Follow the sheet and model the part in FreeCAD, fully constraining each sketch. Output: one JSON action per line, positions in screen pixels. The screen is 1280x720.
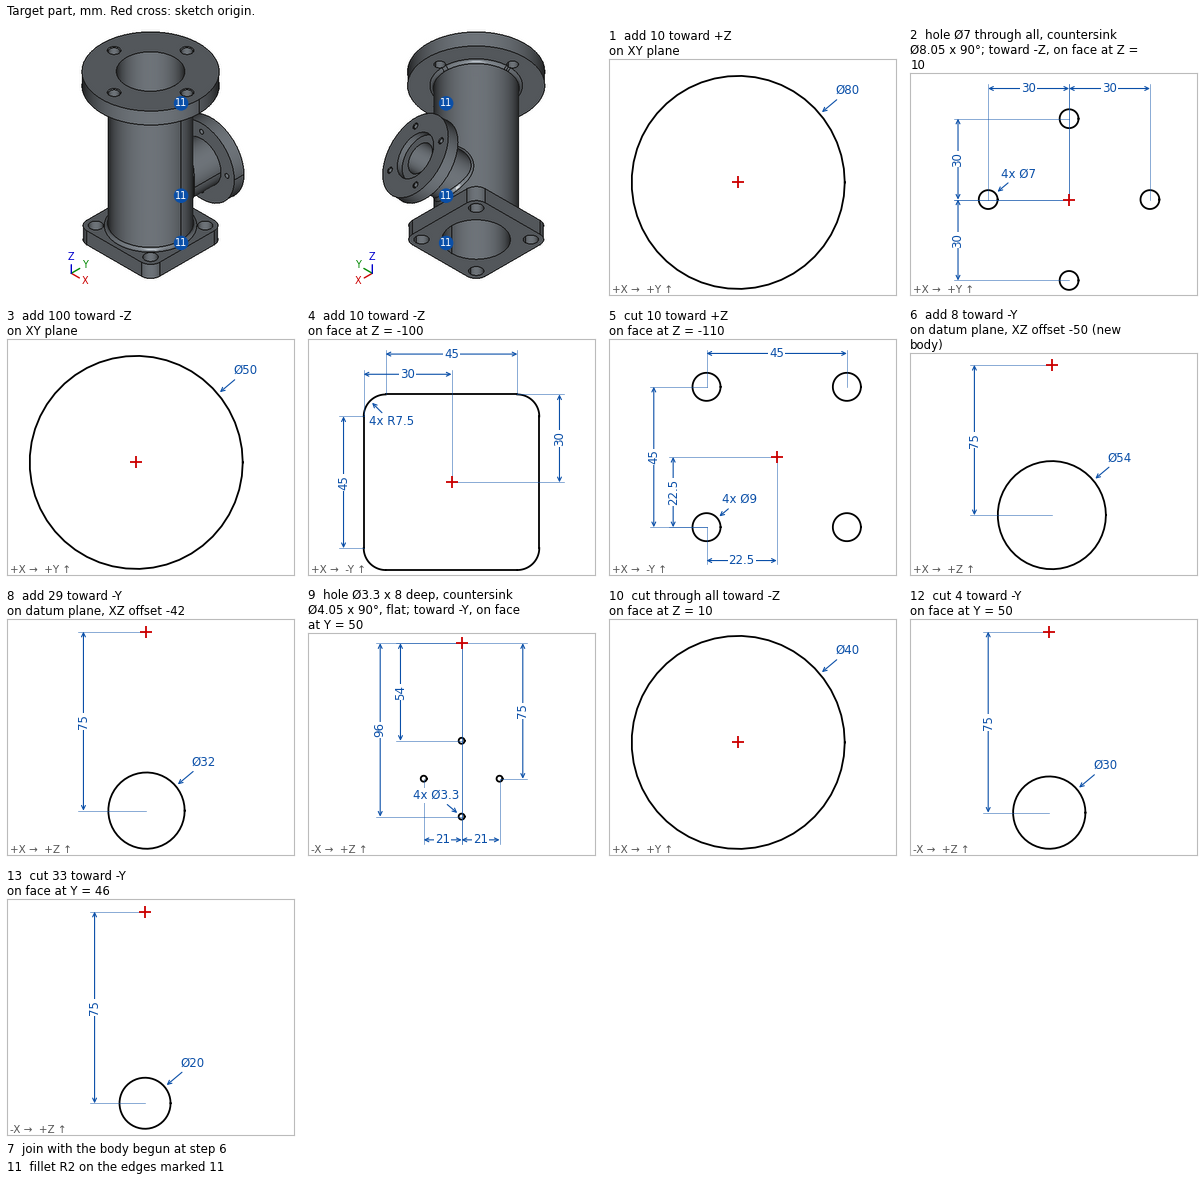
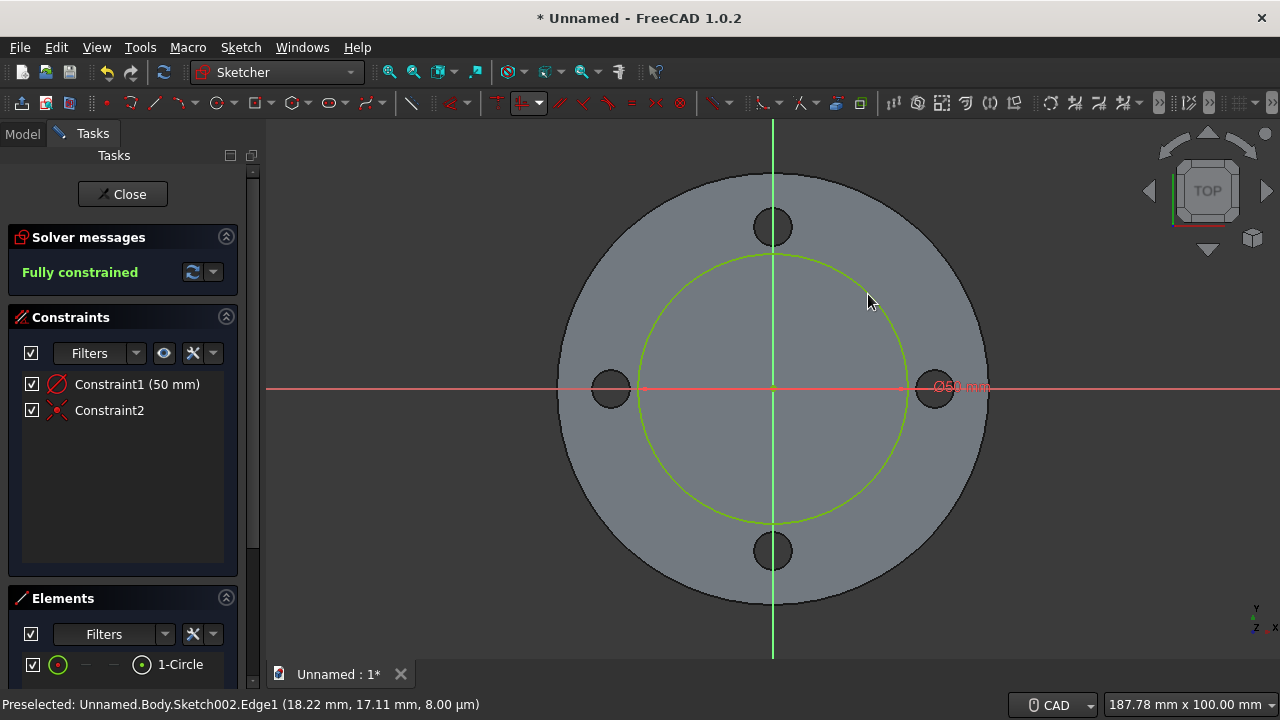
{"action": "left_click", "coordinate": [123, 194]}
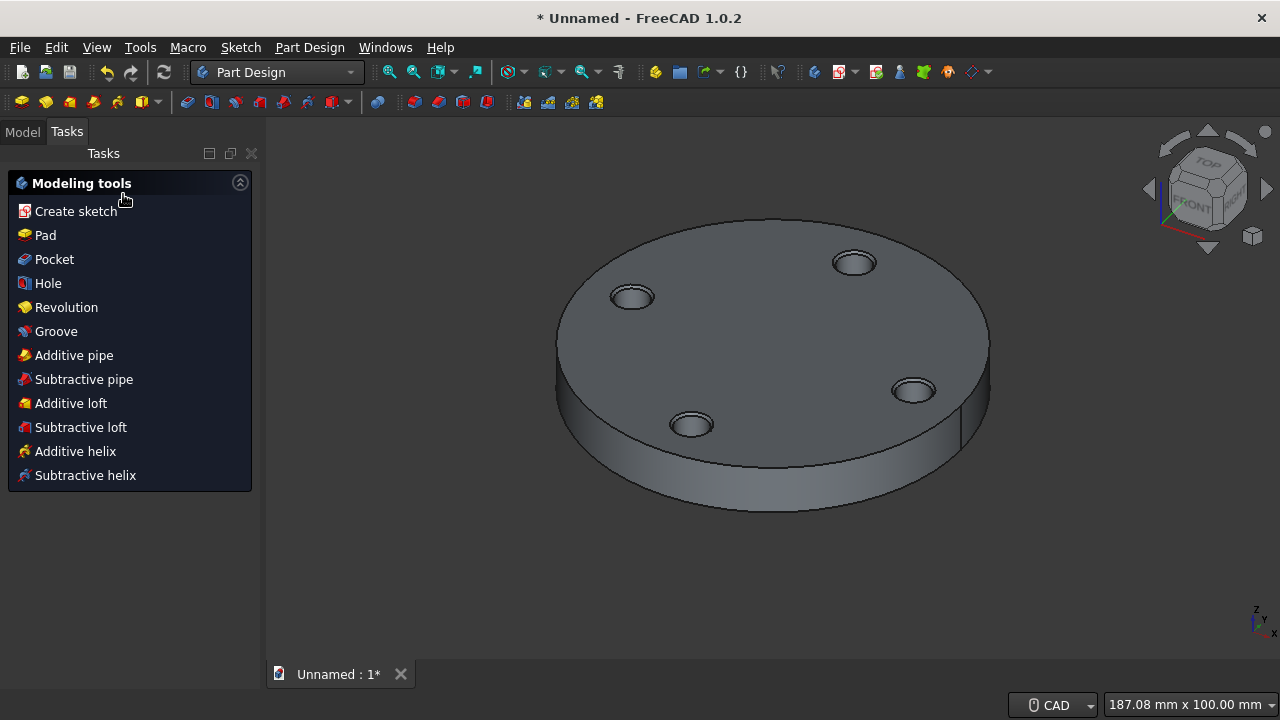
{"action": "left_click", "coordinate": [22, 102]}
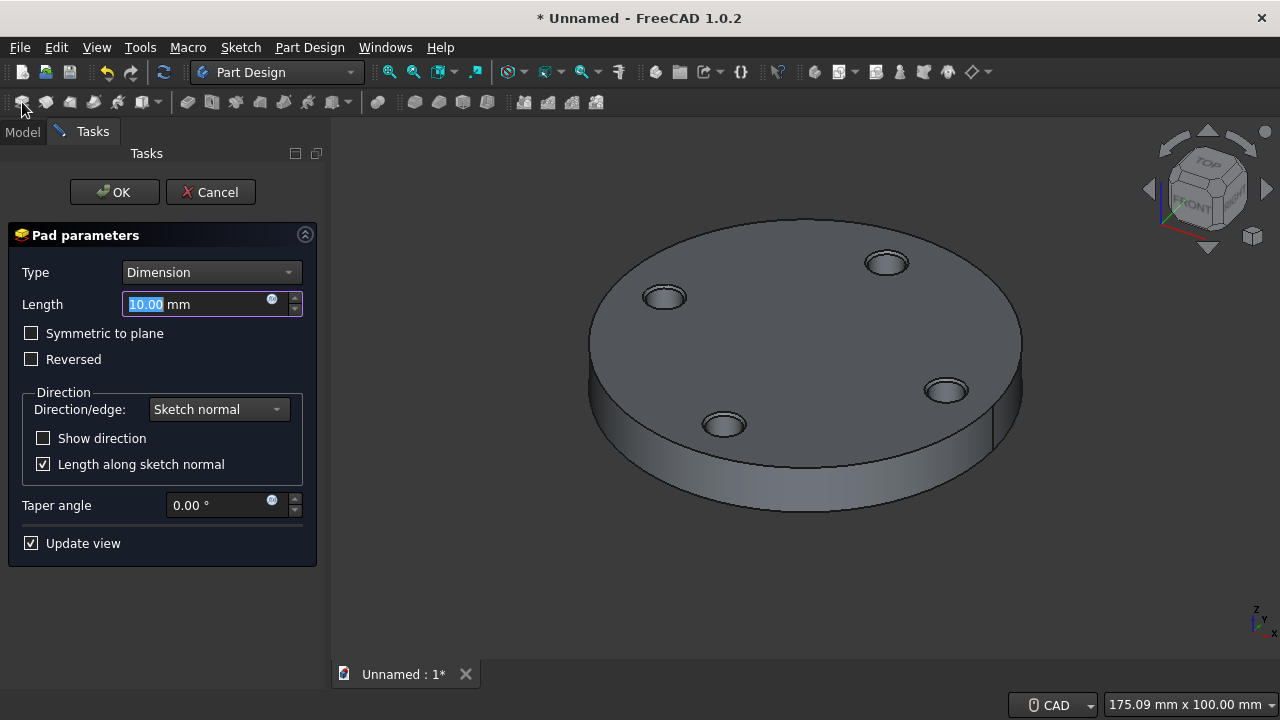
{"action": "type", "text": "100"}
{"action": "key", "text": "Tab"}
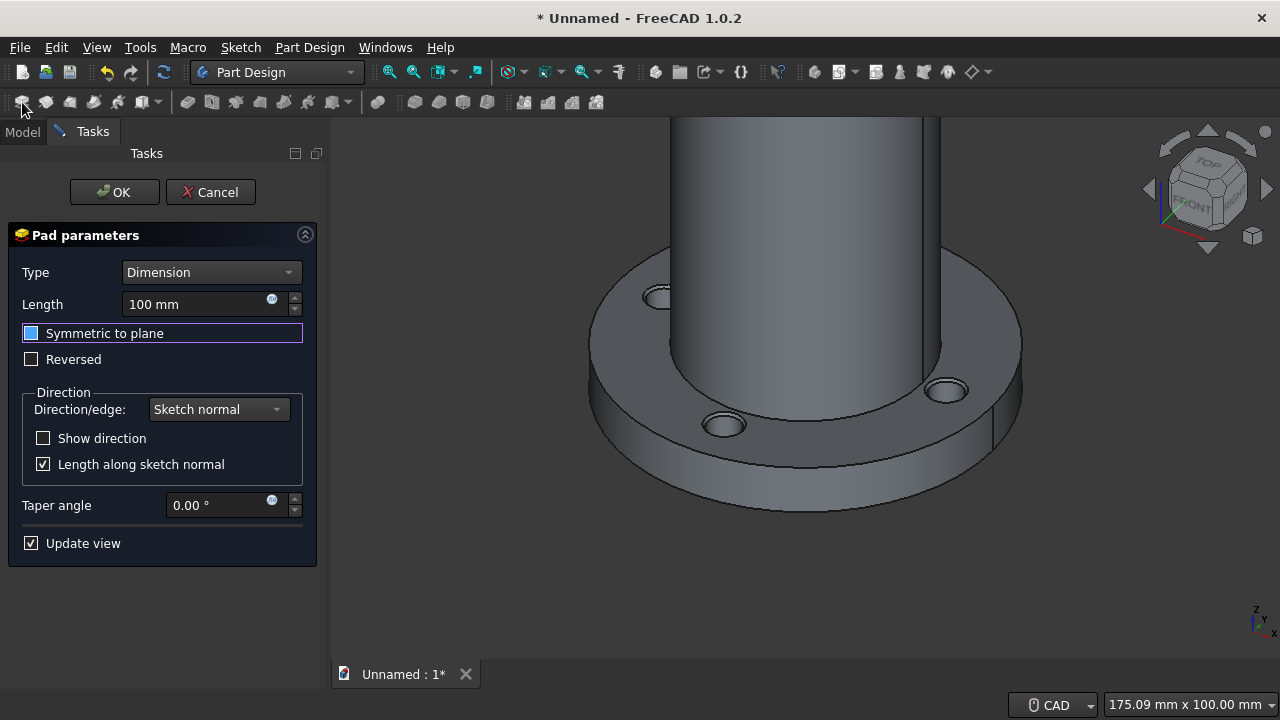
{"action": "left_click", "coordinate": [30, 359]}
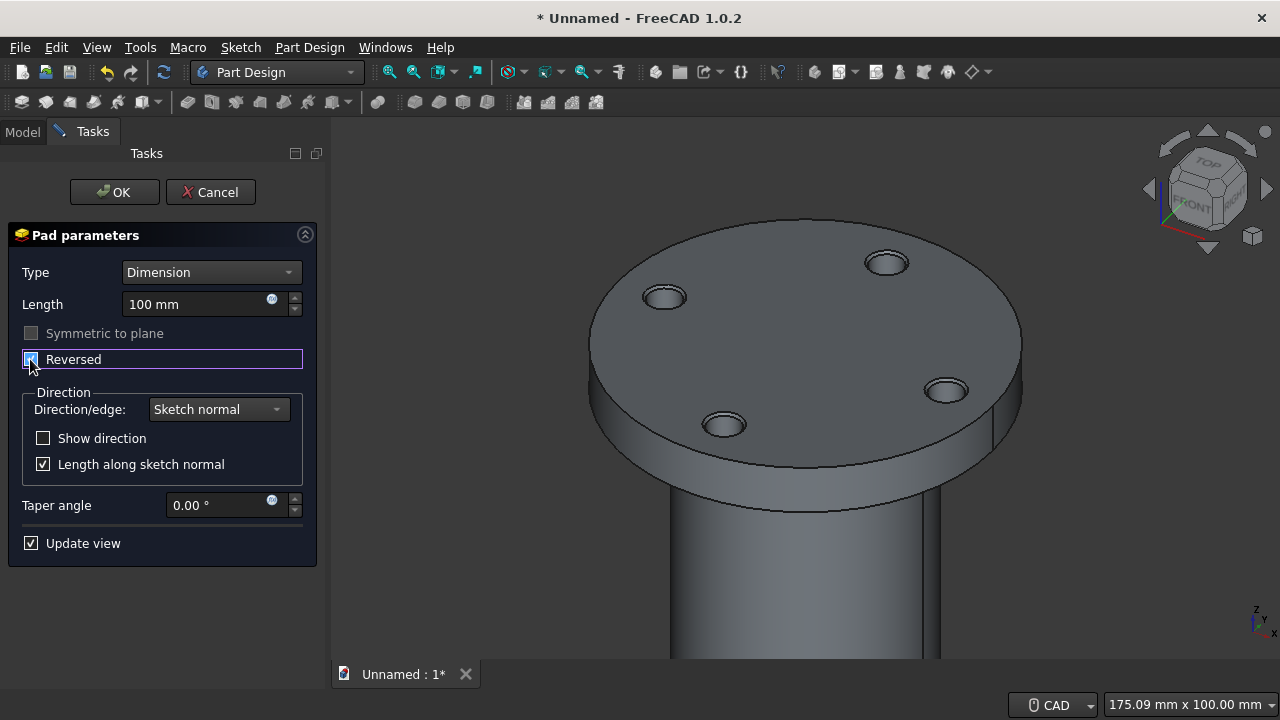
{"action": "left_click", "coordinate": [115, 192]}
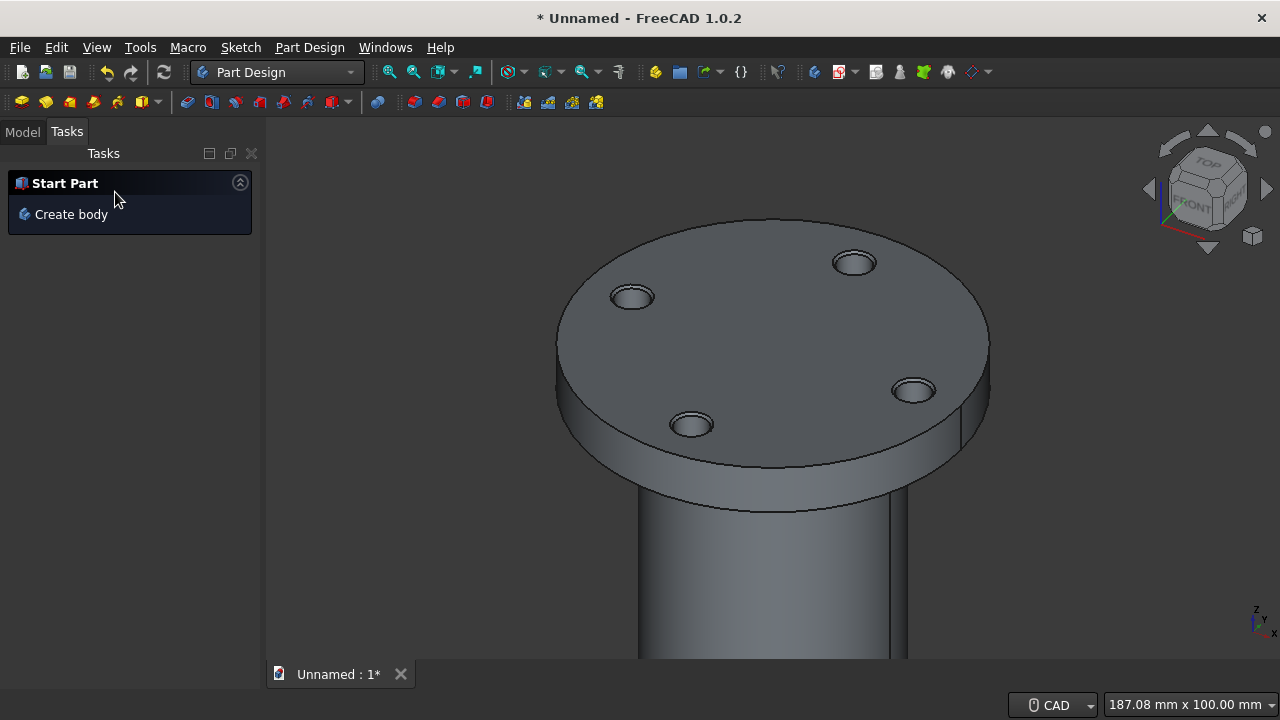
{"action": "left_click", "coordinate": [390, 72]}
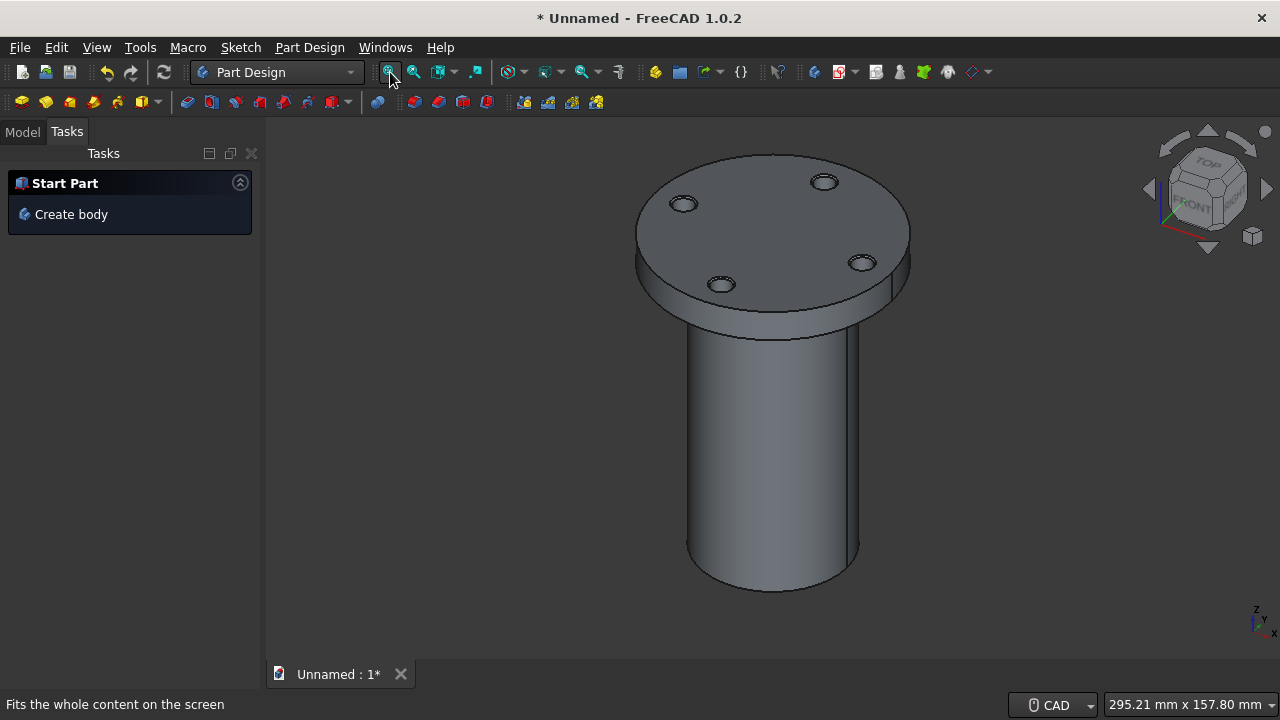
{"action": "key", "text": "5"}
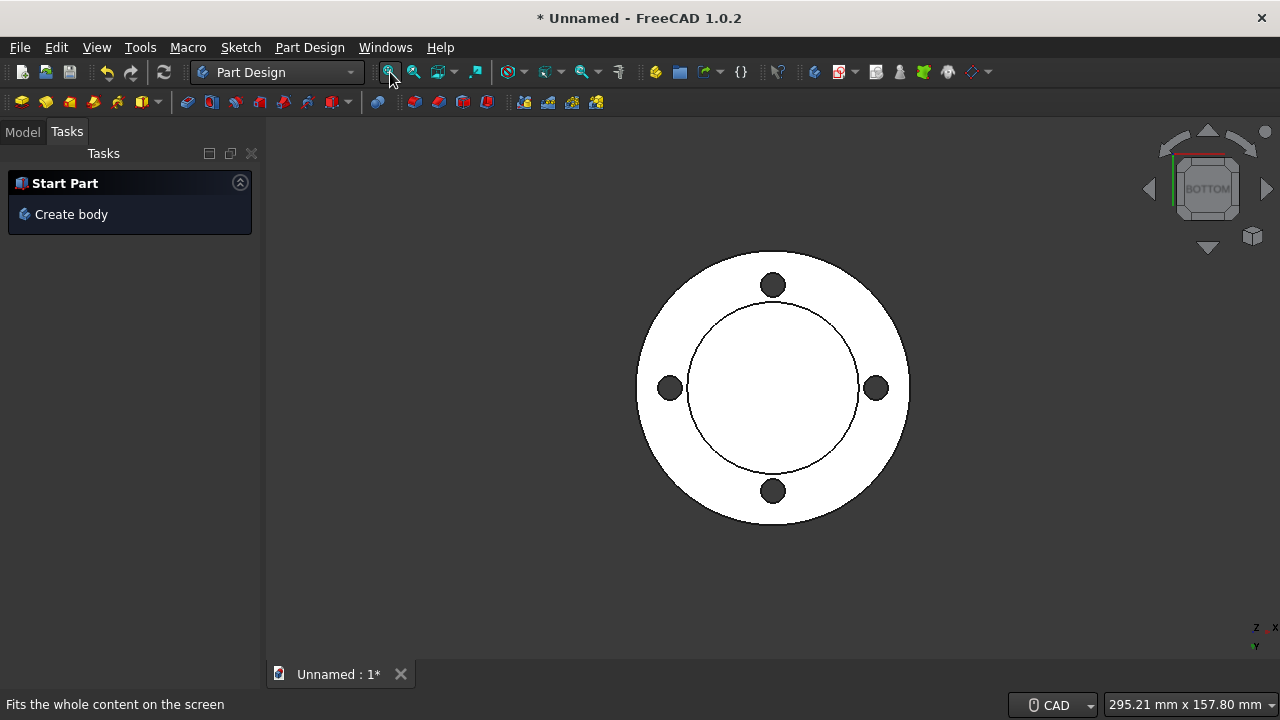
{"action": "left_click", "coordinate": [773, 387]}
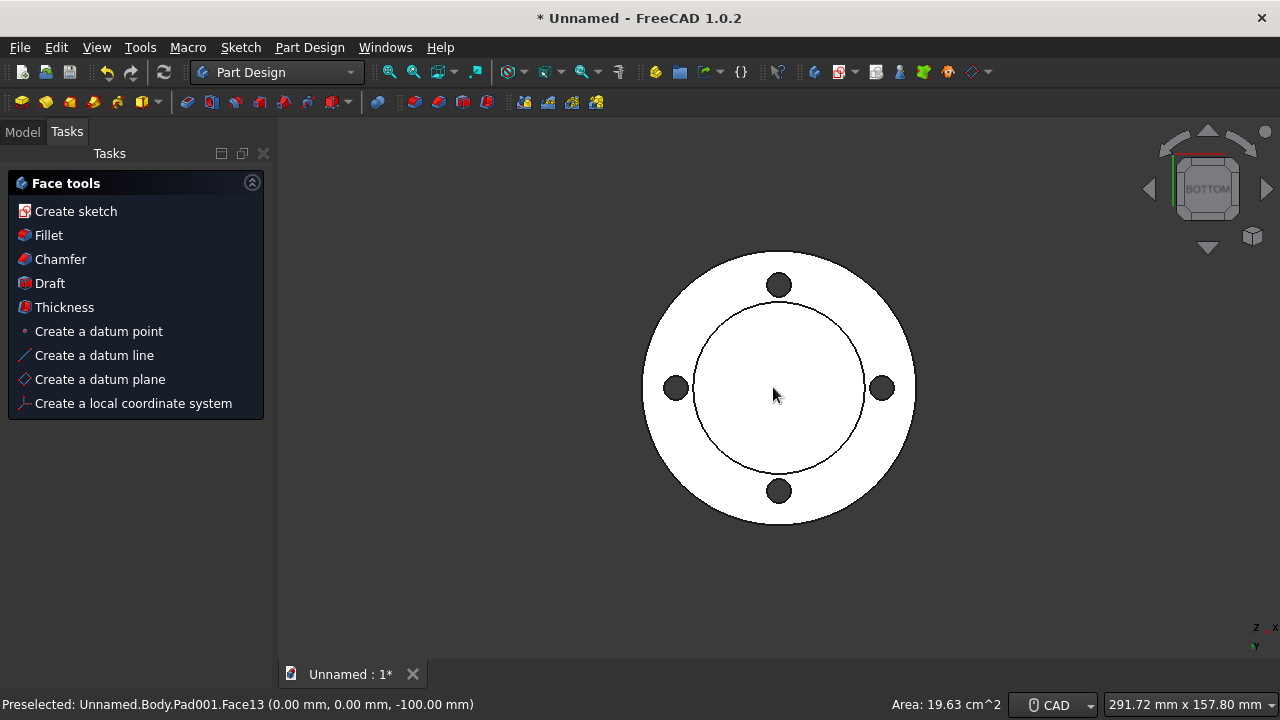
{"action": "left_click", "coordinate": [840, 72]}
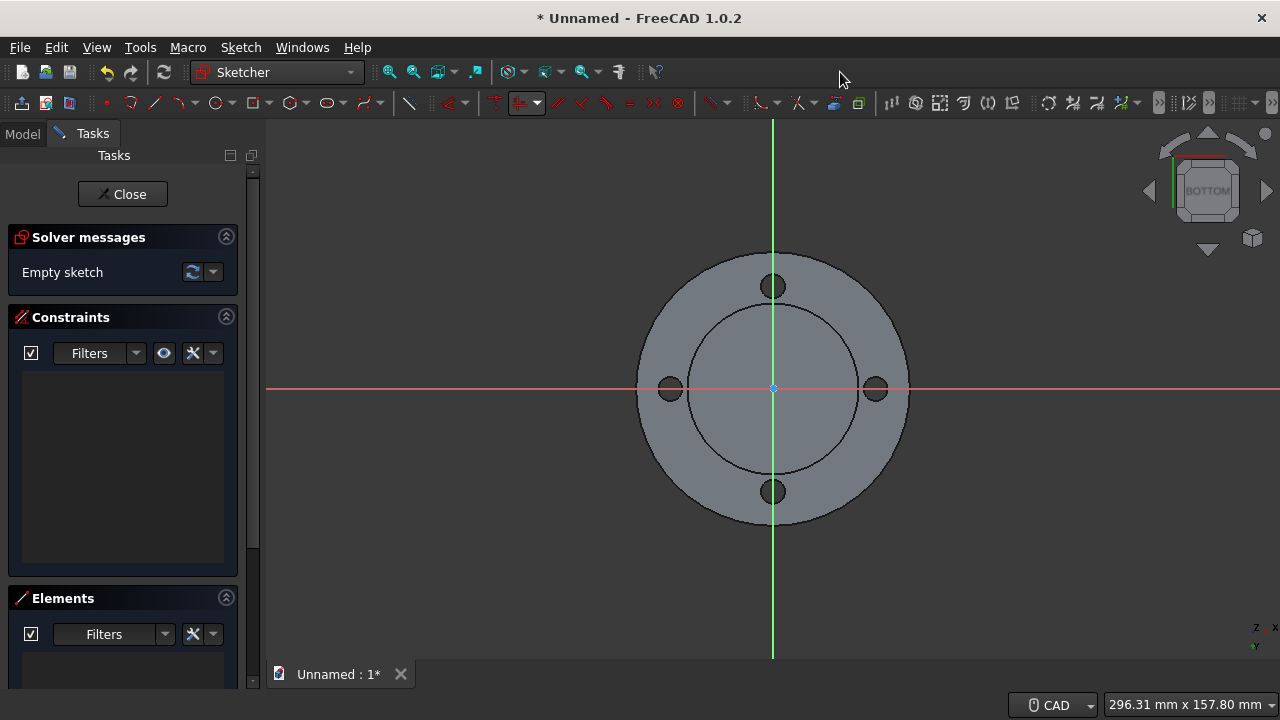
{"action": "scroll", "coordinate": [856, 389], "scroll_direction": "up", "scroll_amount": 3}